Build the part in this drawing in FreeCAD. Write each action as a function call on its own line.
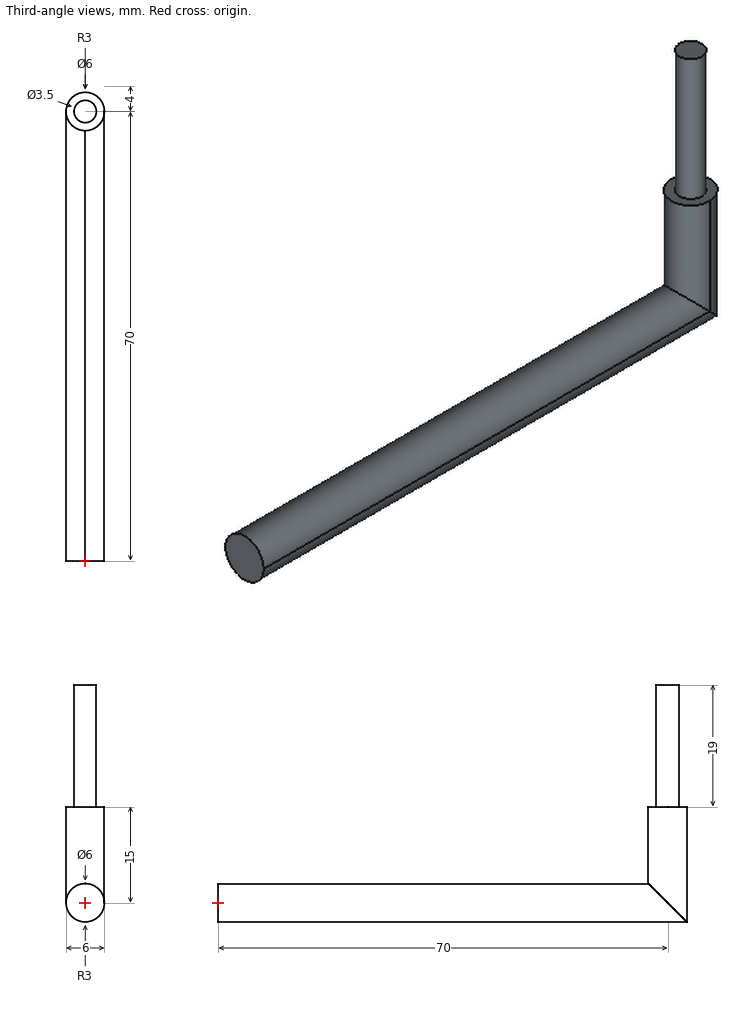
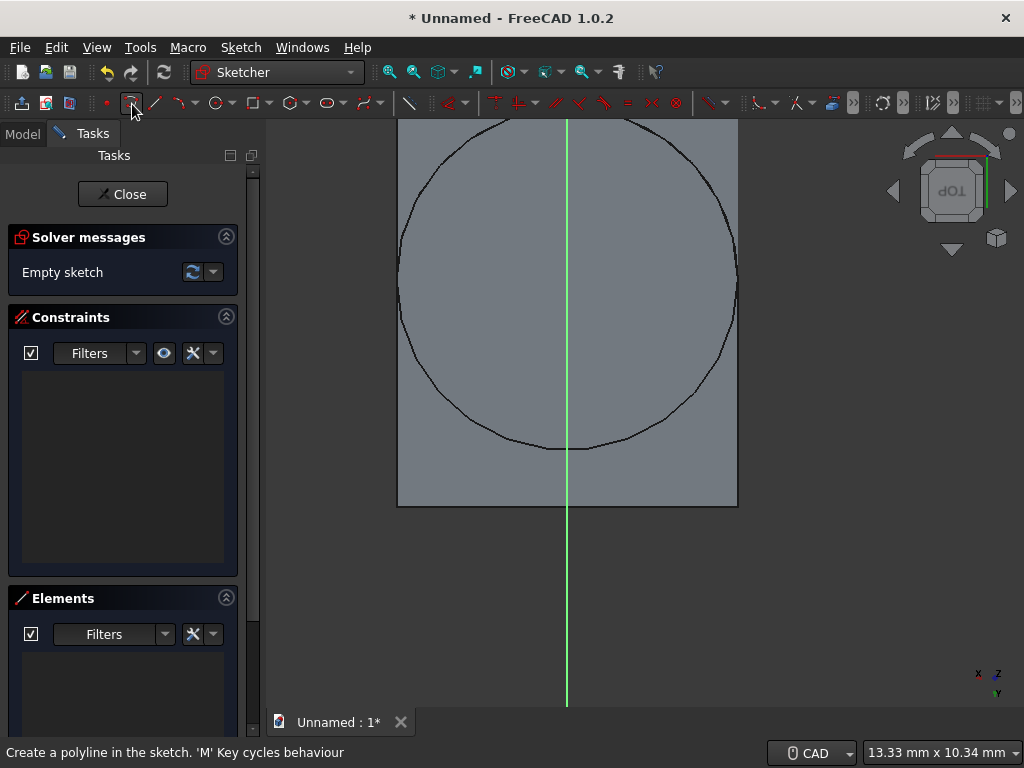
click(397, 279)
click(397, 507)
click(738, 507)
click(738, 279)
right_click(738, 279)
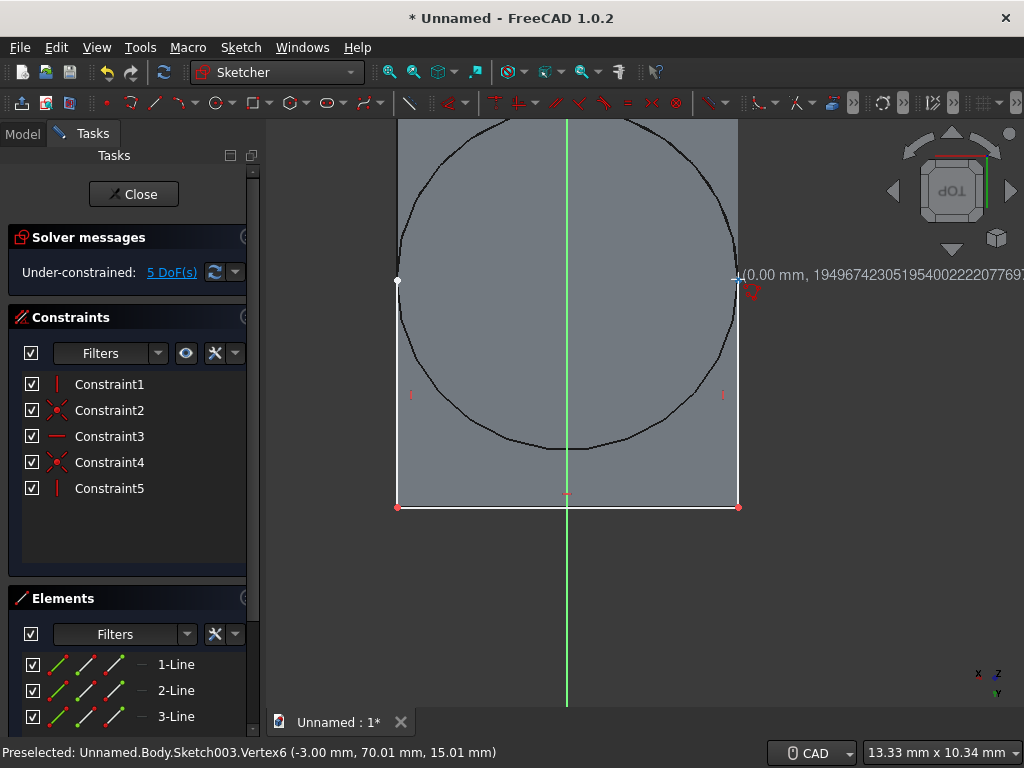
key(g)
key(3)
key(a)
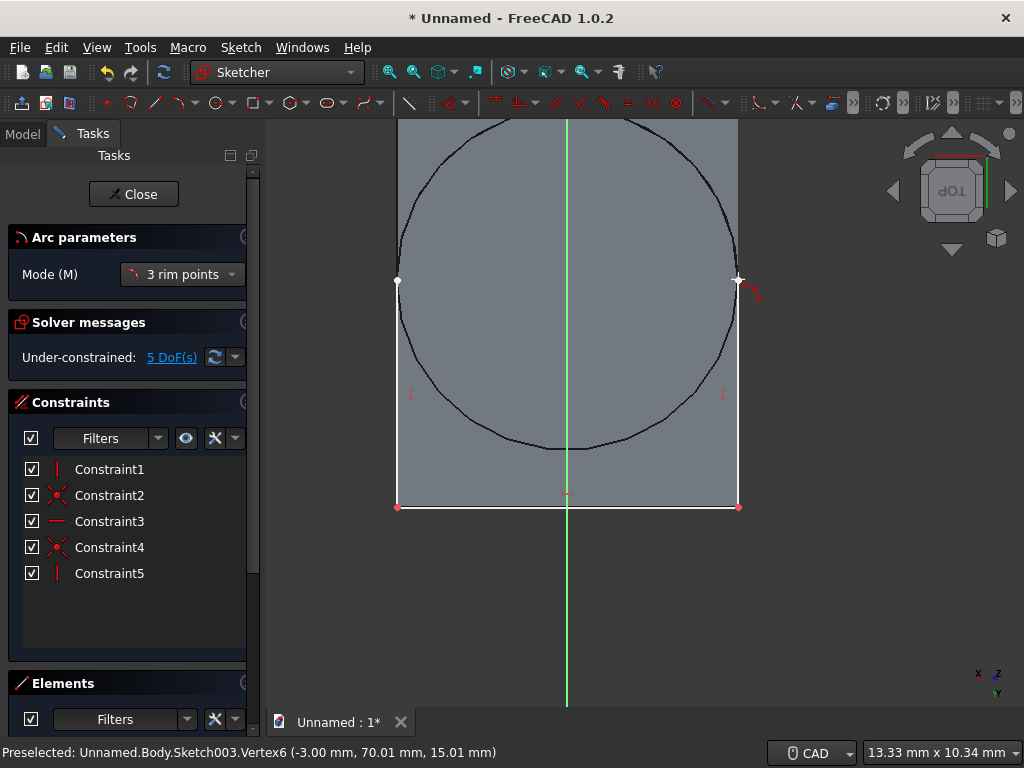
click(738, 280)
click(397, 280)
click(515, 442)
key(Escape)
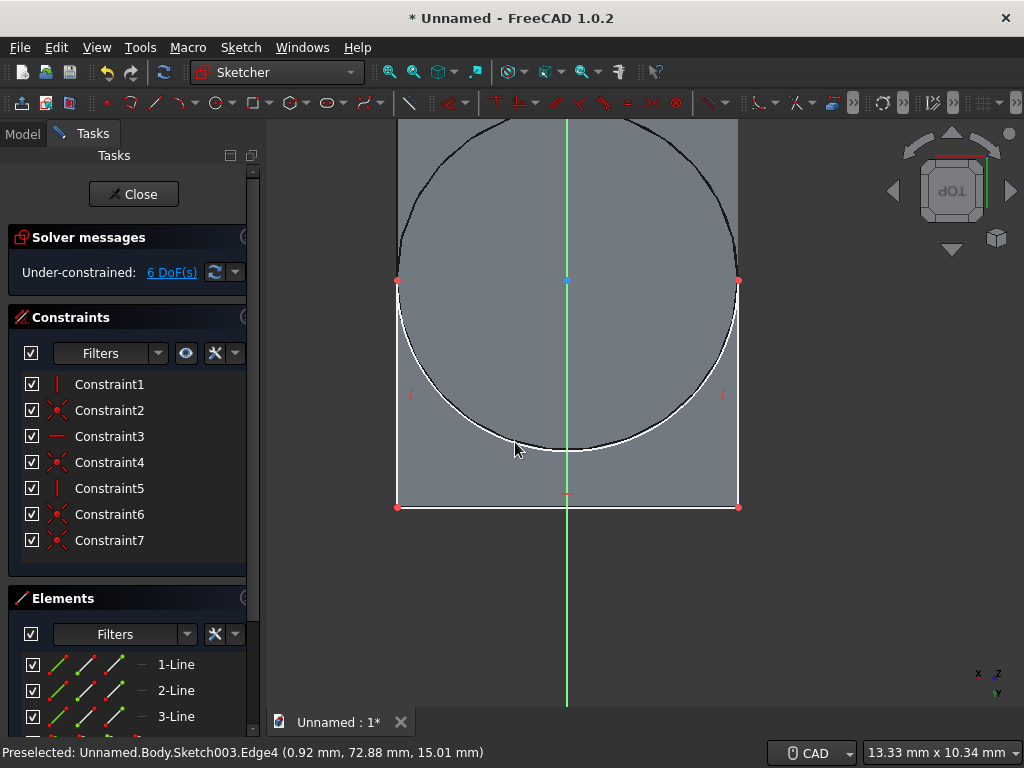
click(397, 348)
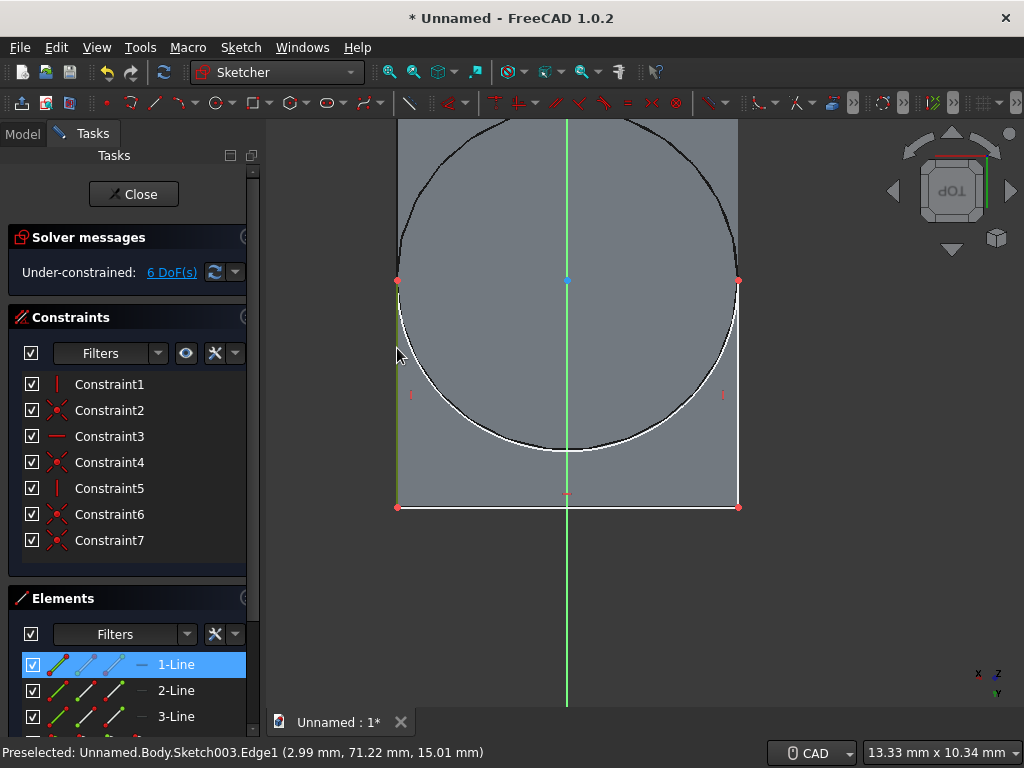
click(467, 419)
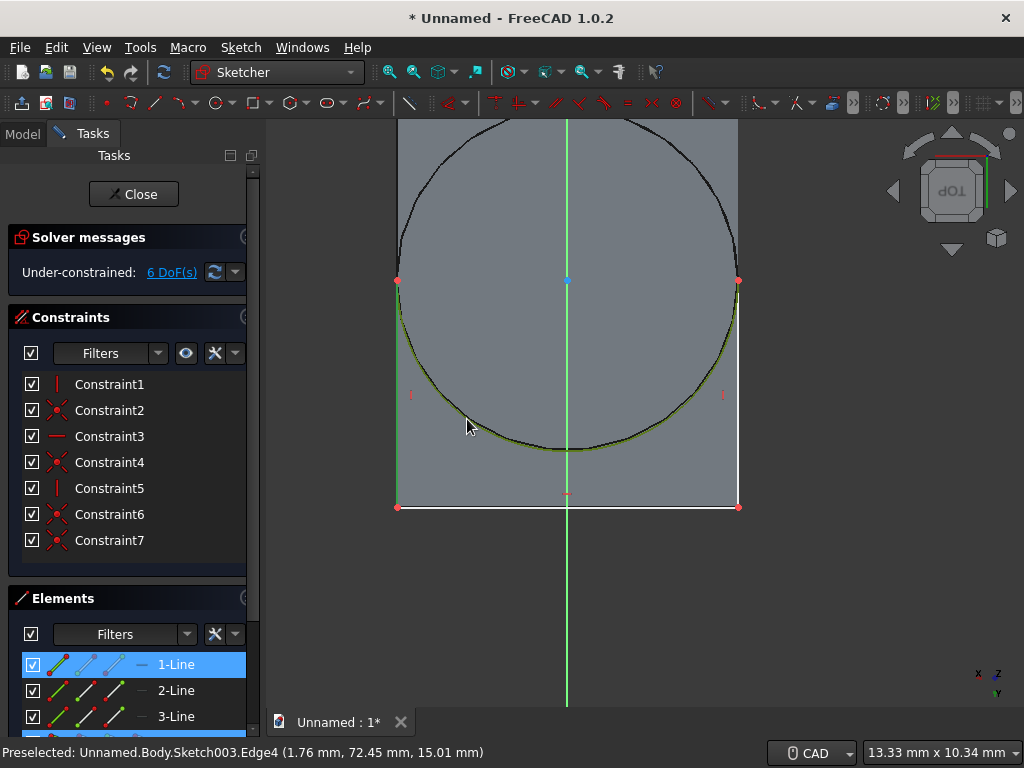
click(604, 104)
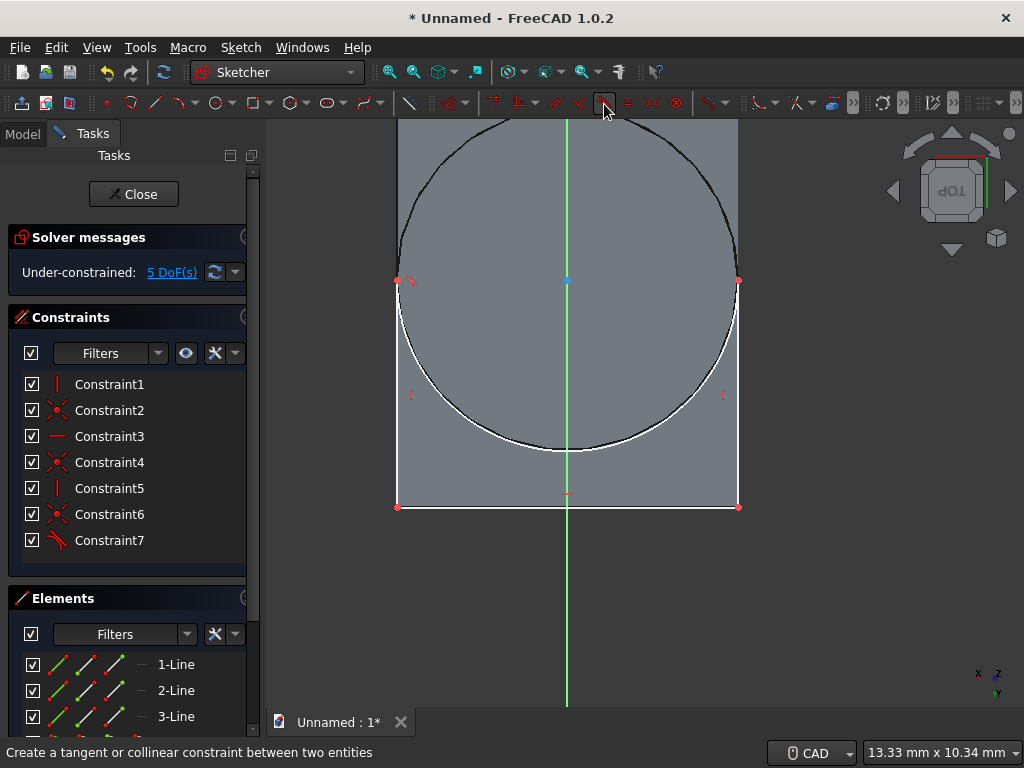
click(738, 440)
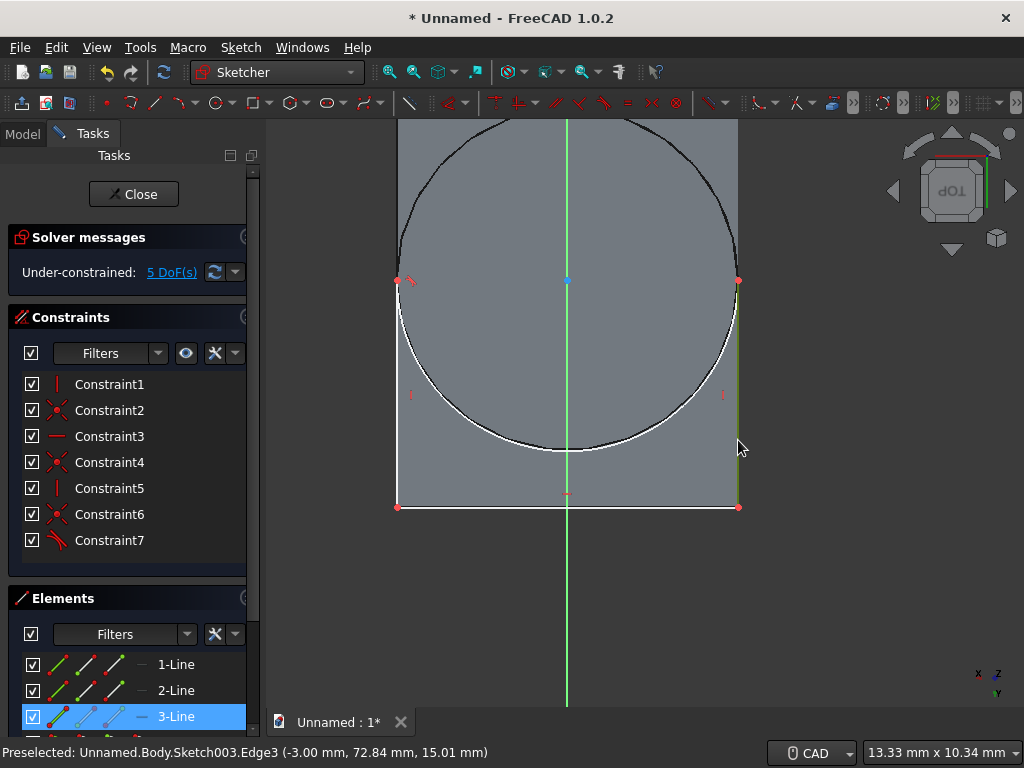
click(467, 419)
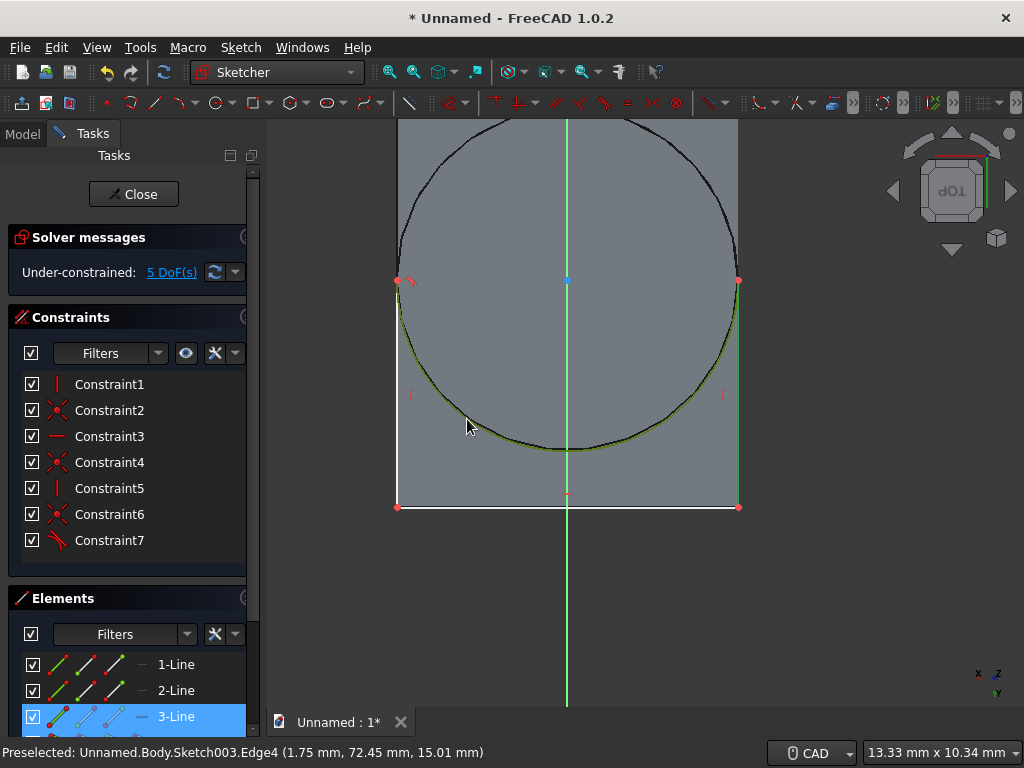
key(t)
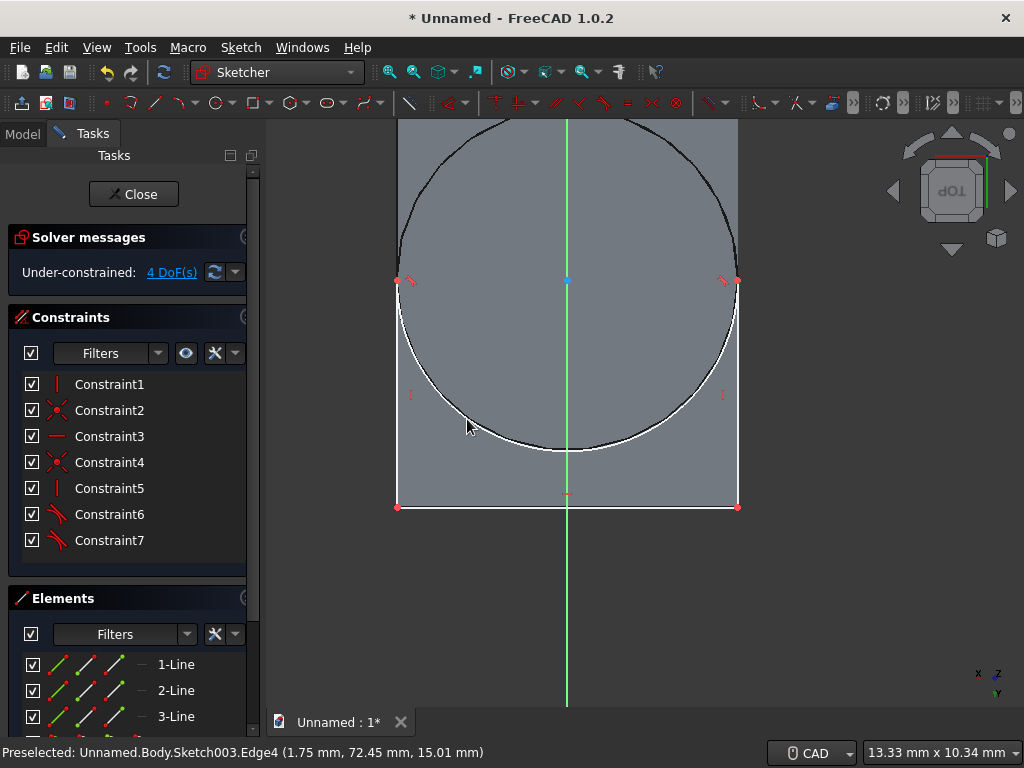
click(567, 281)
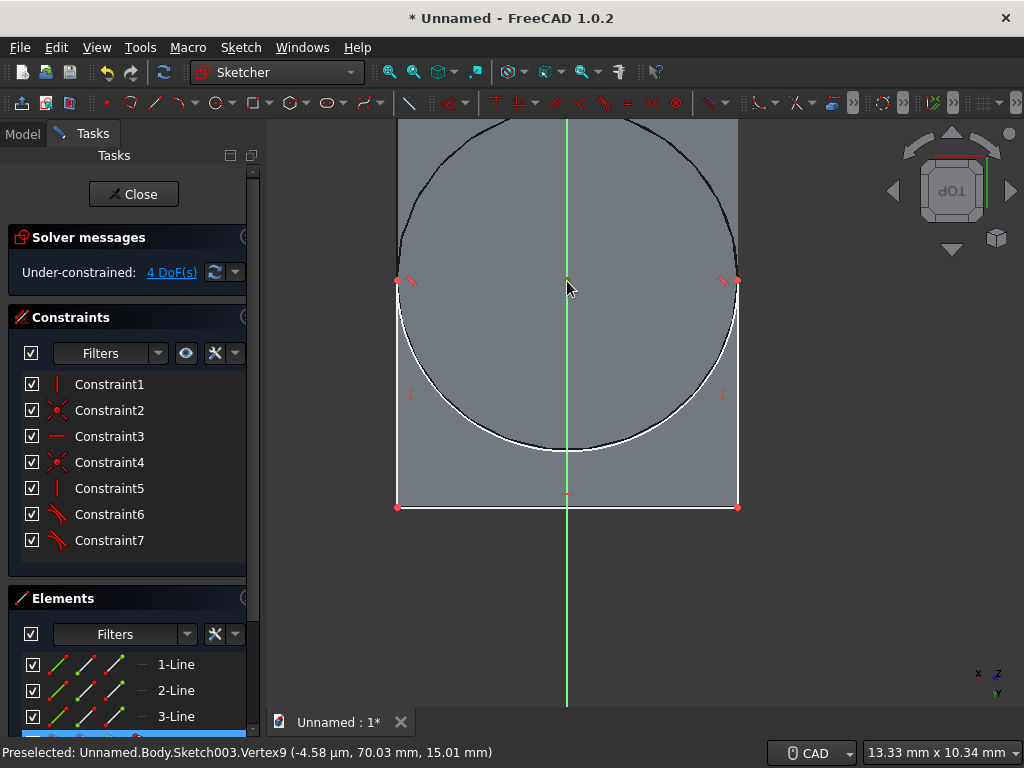
click(567, 641)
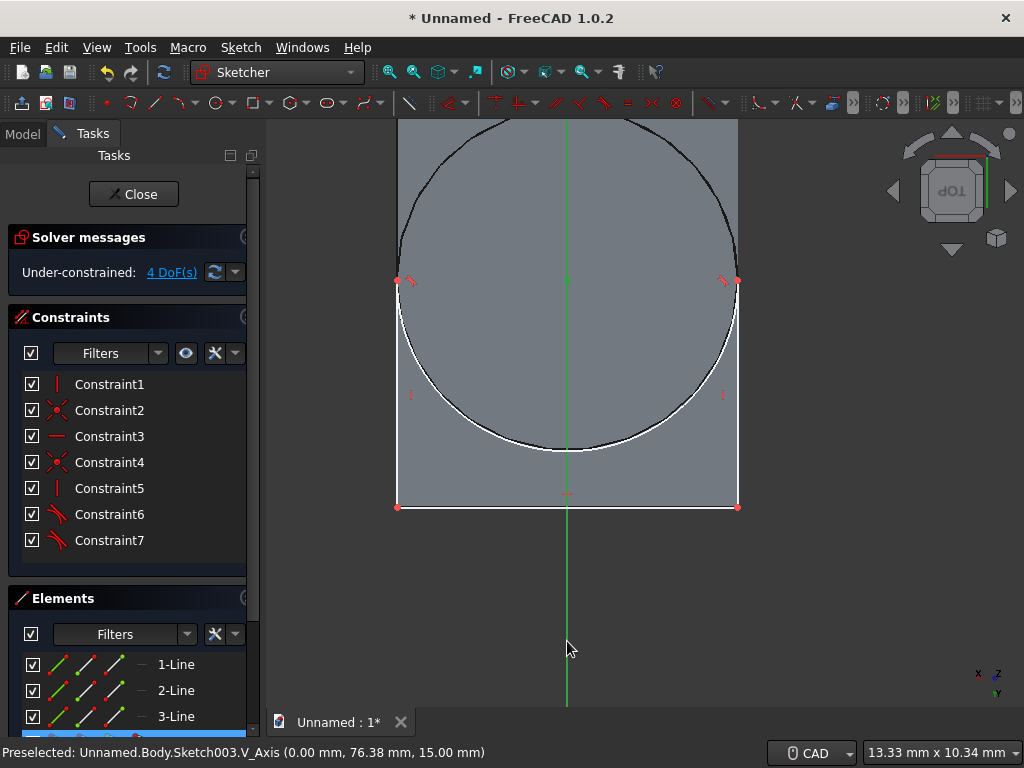
click(496, 104)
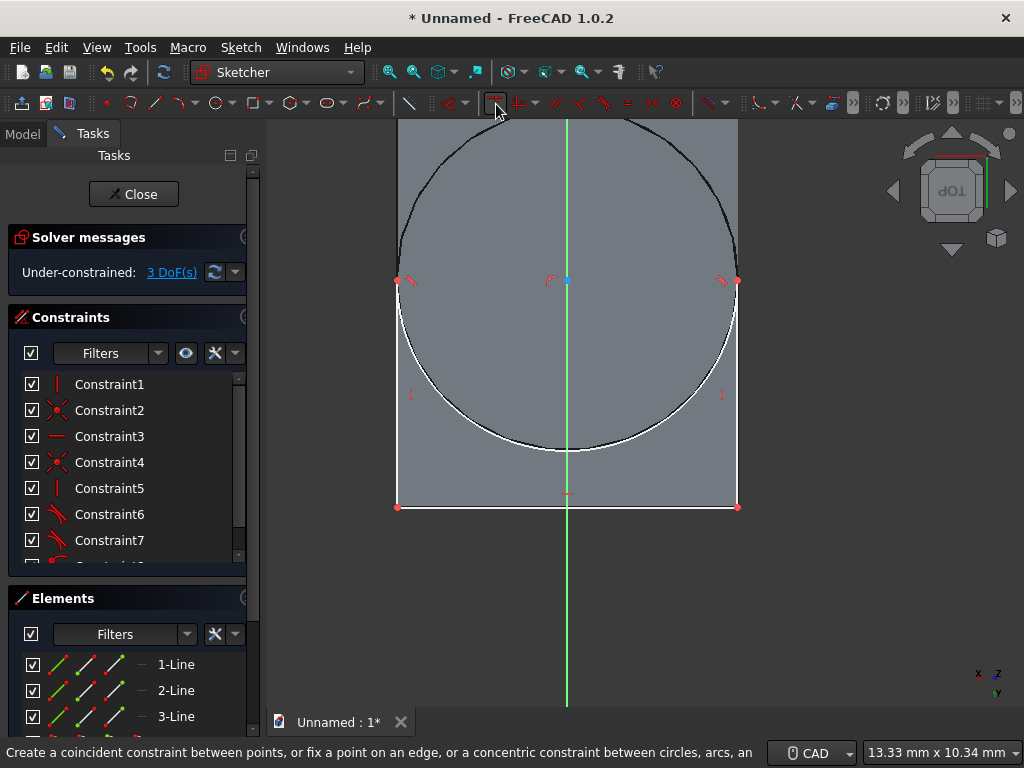
click(448, 104)